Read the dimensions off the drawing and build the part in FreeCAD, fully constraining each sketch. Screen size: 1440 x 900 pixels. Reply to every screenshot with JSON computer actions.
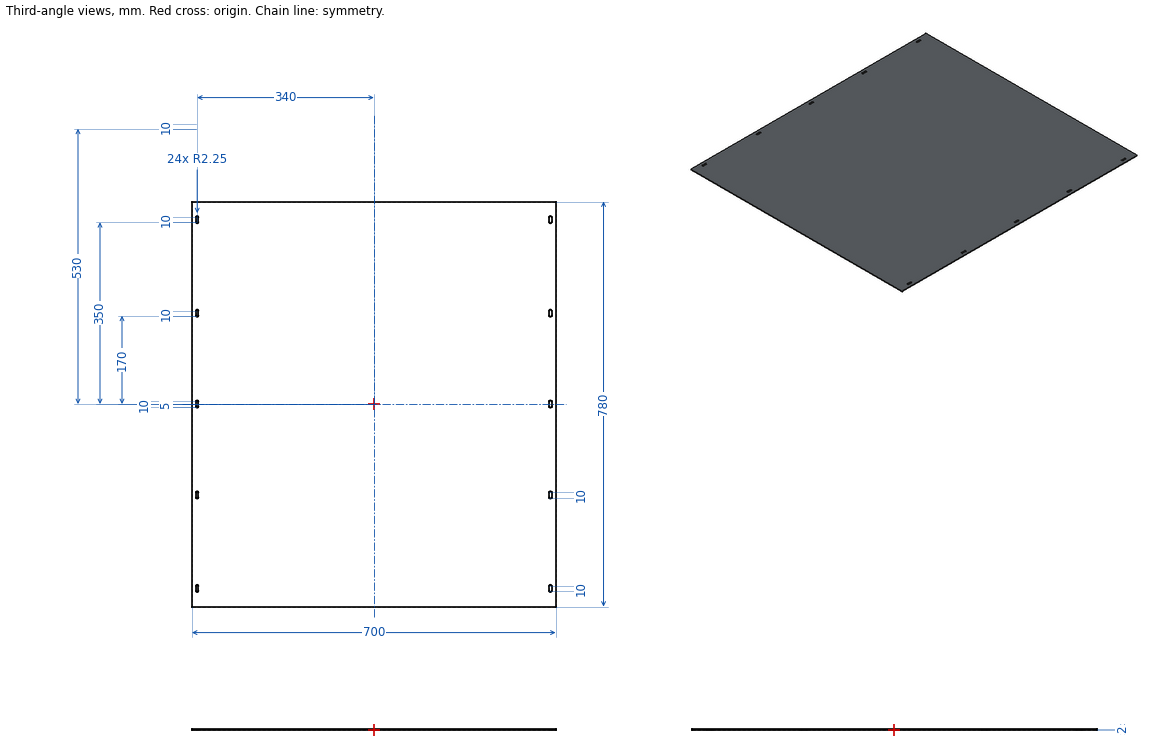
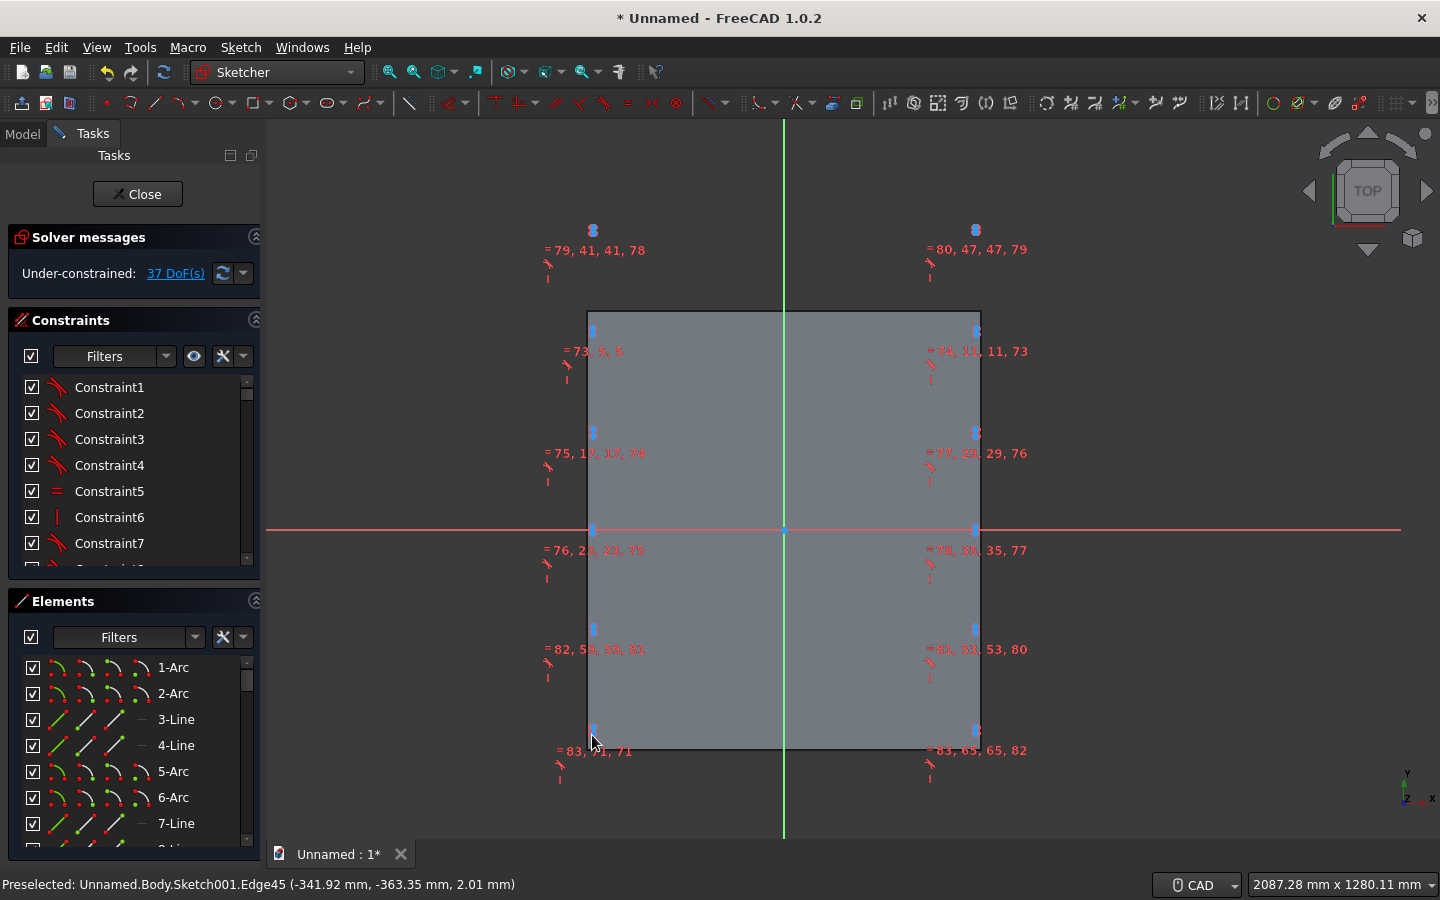
{"action": "scroll", "coordinate": [593, 335], "scroll_direction": "up", "scroll_amount": 12}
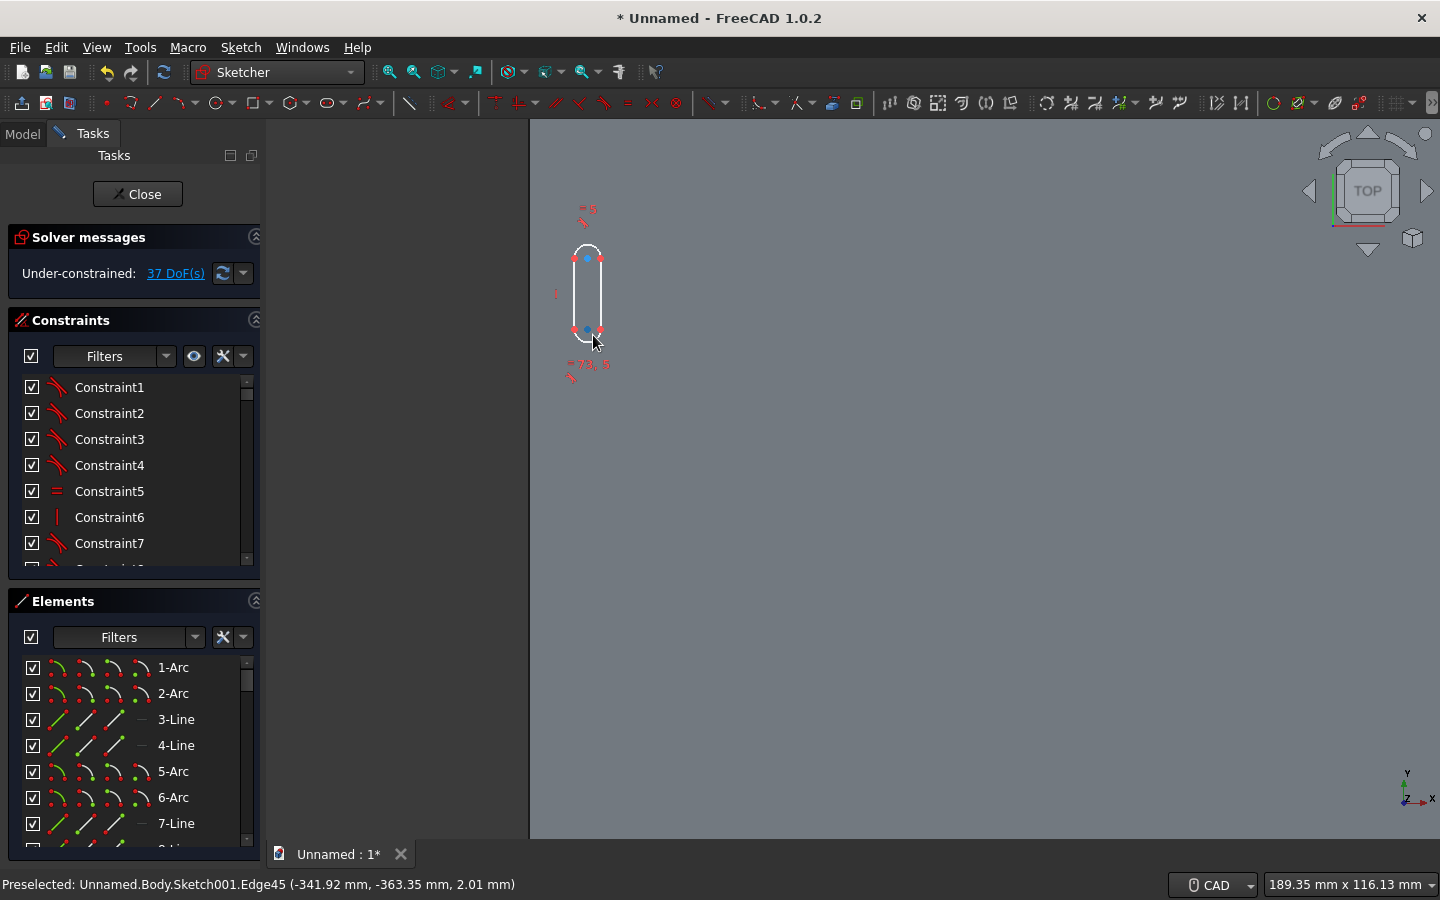
{"action": "left_click", "coordinate": [588, 329]}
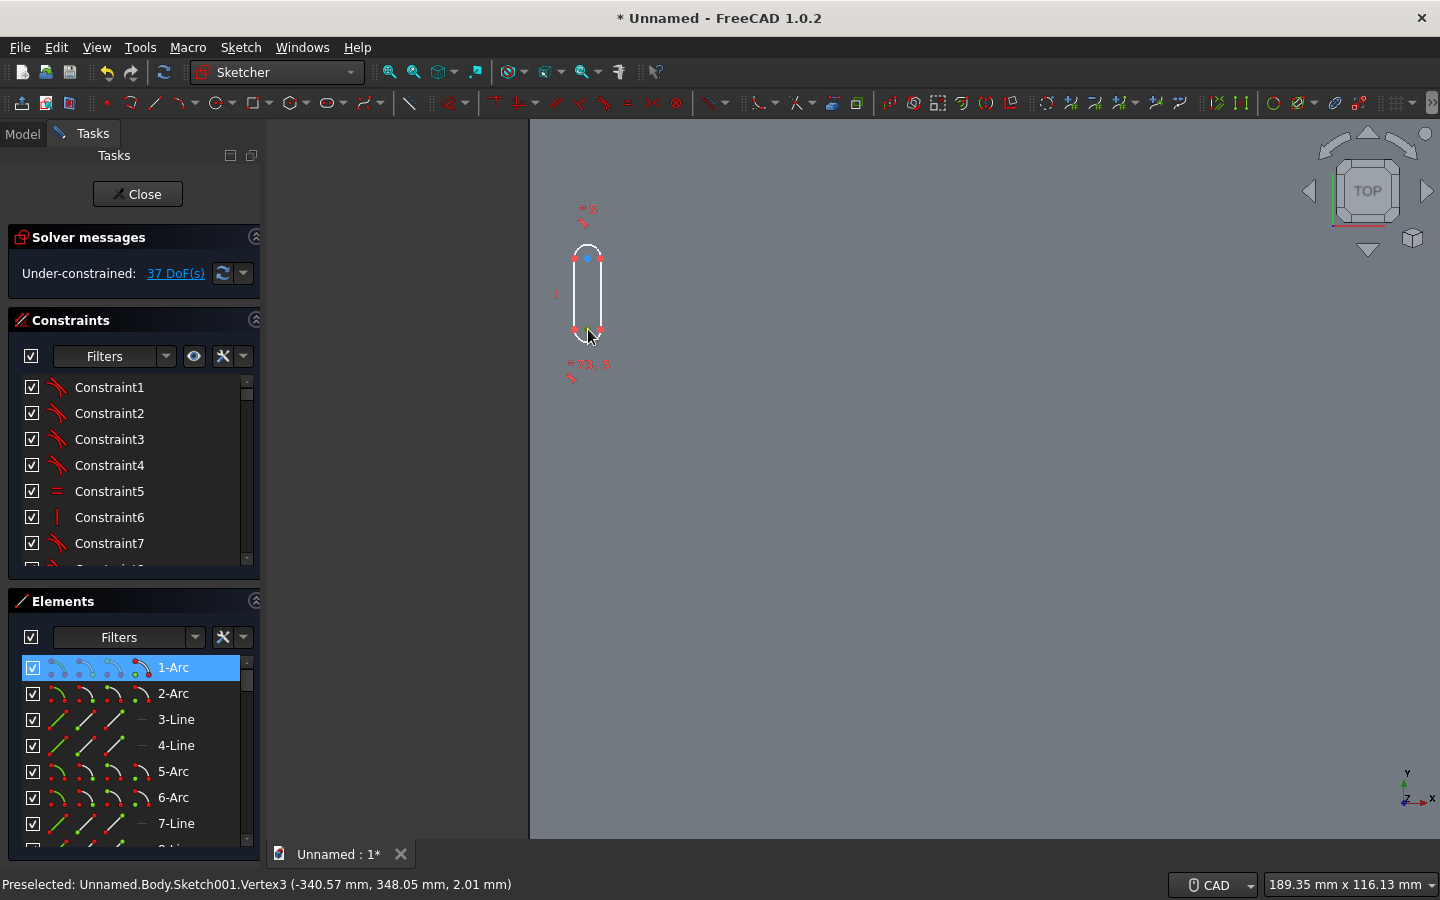
{"action": "scroll", "coordinate": [593, 334], "scroll_direction": "down", "scroll_amount": 12}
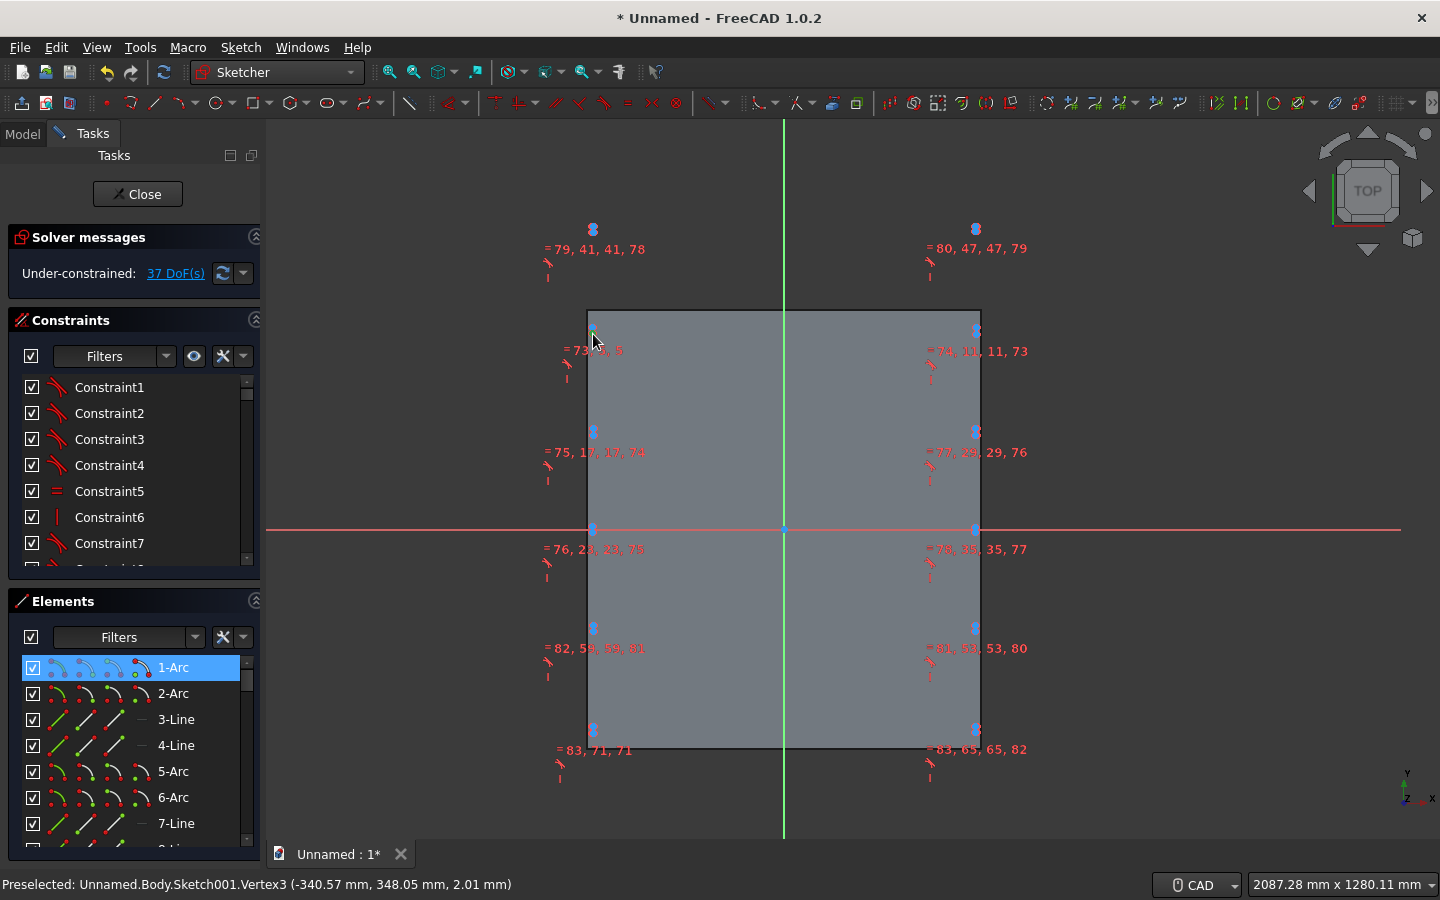
{"action": "scroll", "coordinate": [976, 334], "scroll_direction": "up", "scroll_amount": 12}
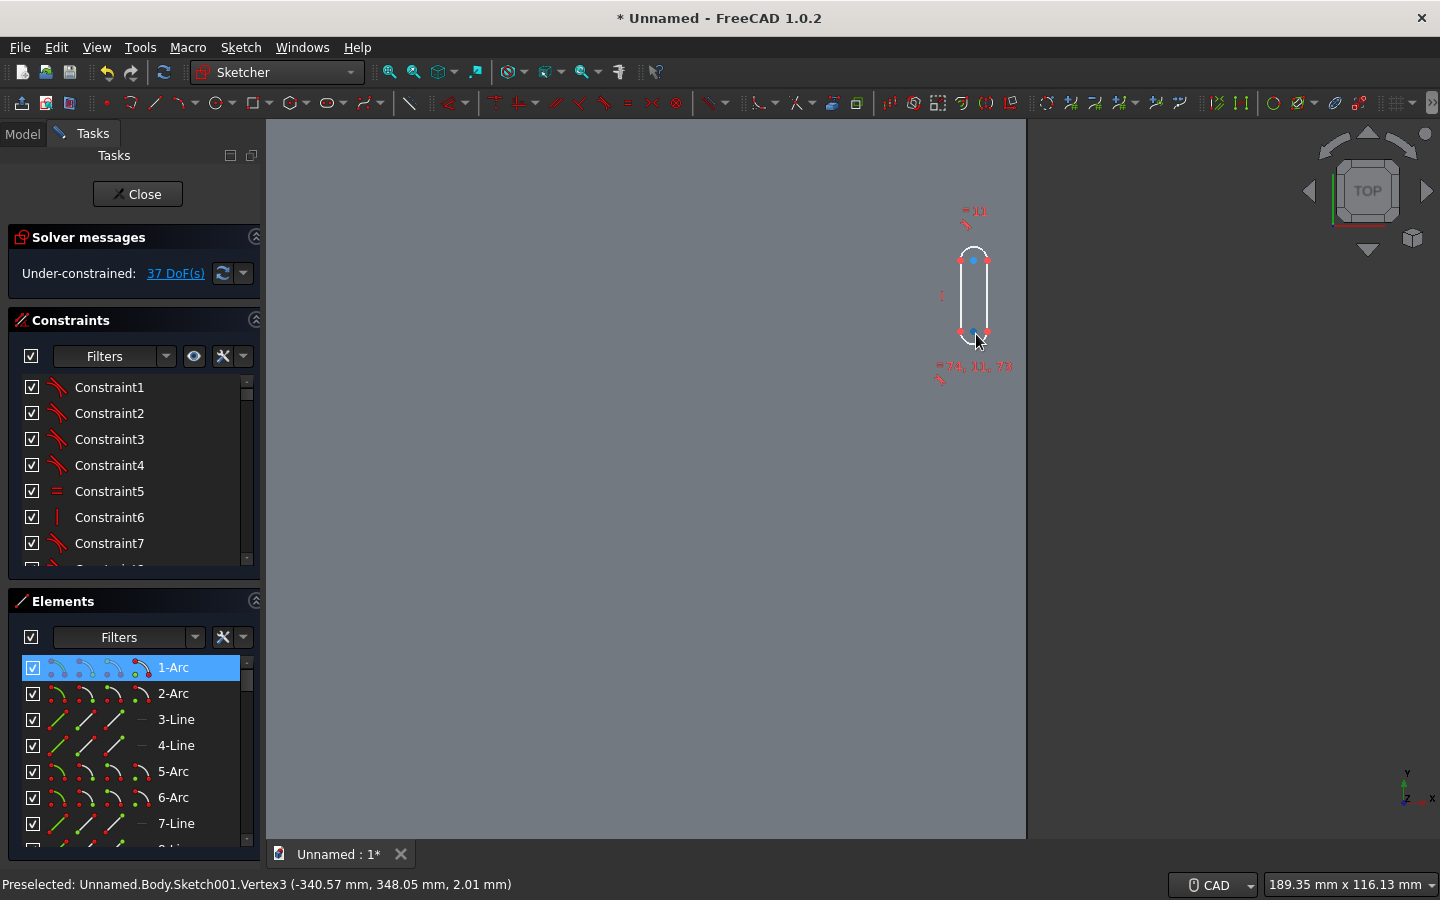
{"action": "left_click", "coordinate": [974, 331]}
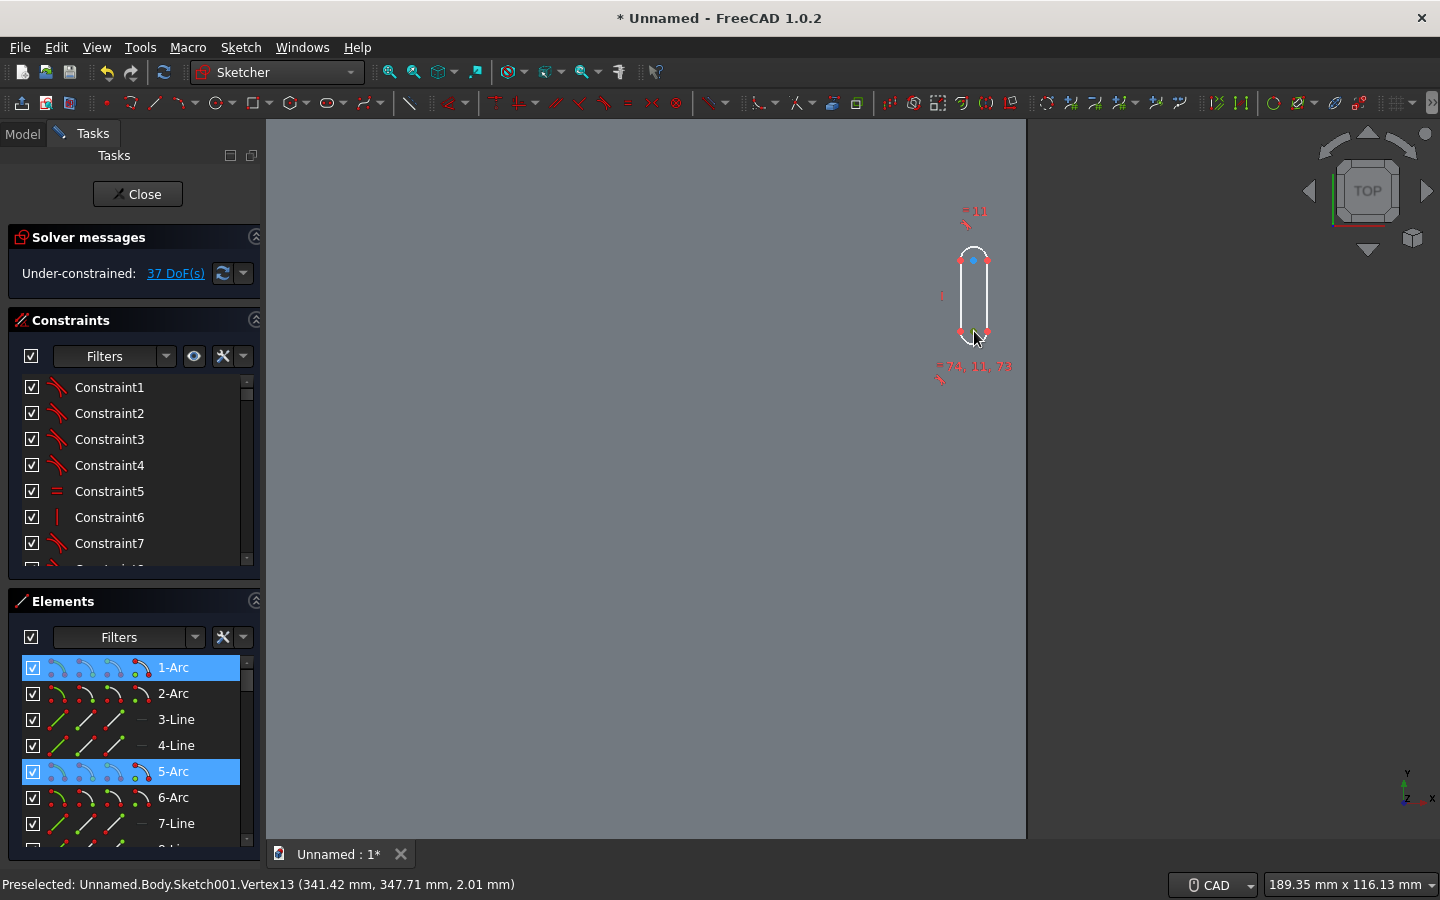
{"action": "scroll", "coordinate": [977, 334], "scroll_direction": "down", "scroll_amount": 12}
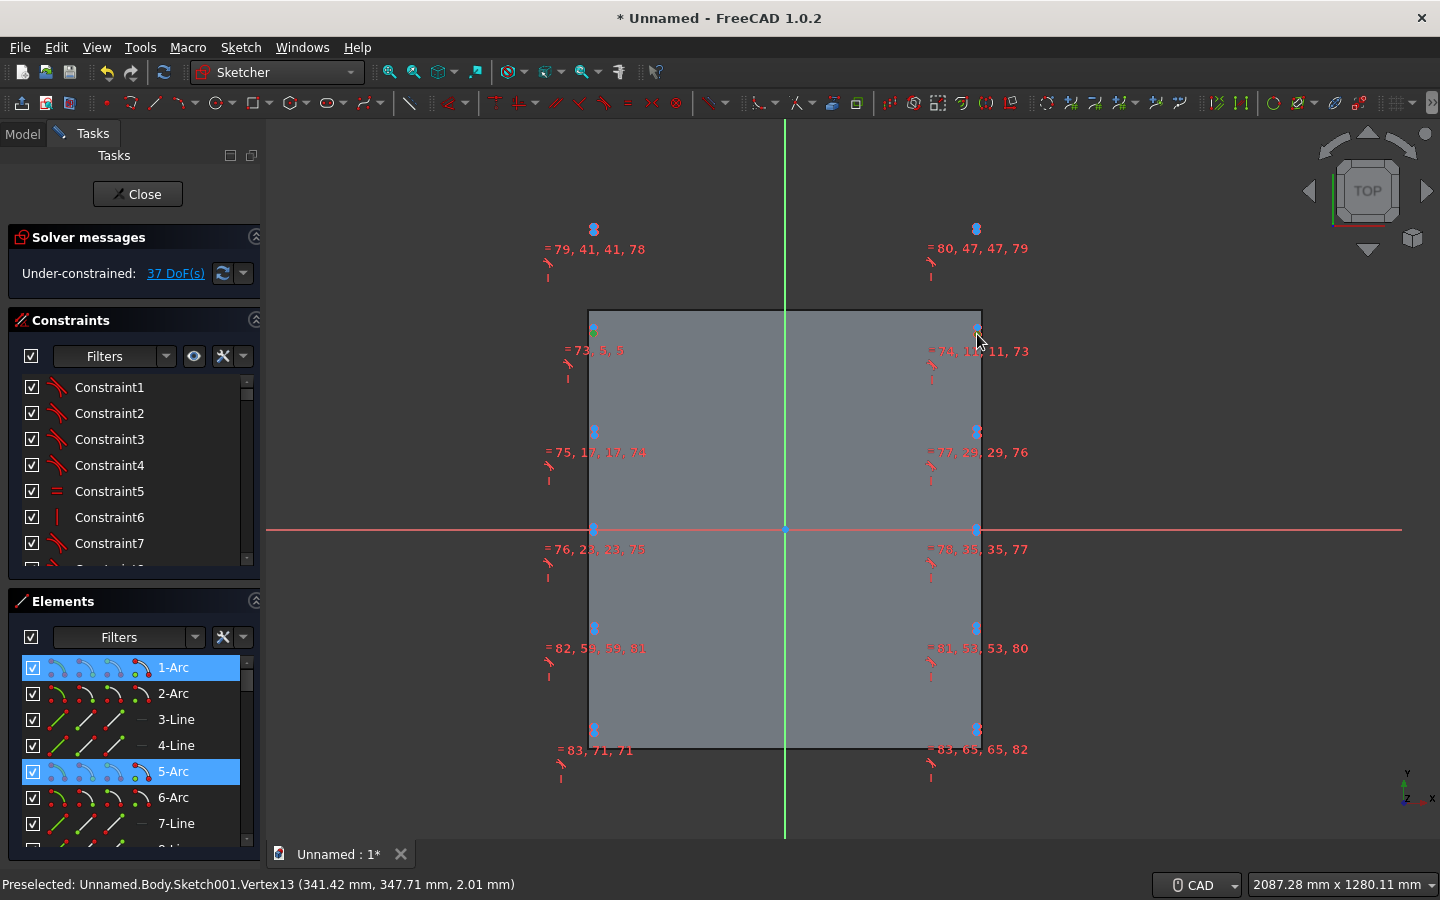
{"action": "left_click", "coordinate": [785, 764]}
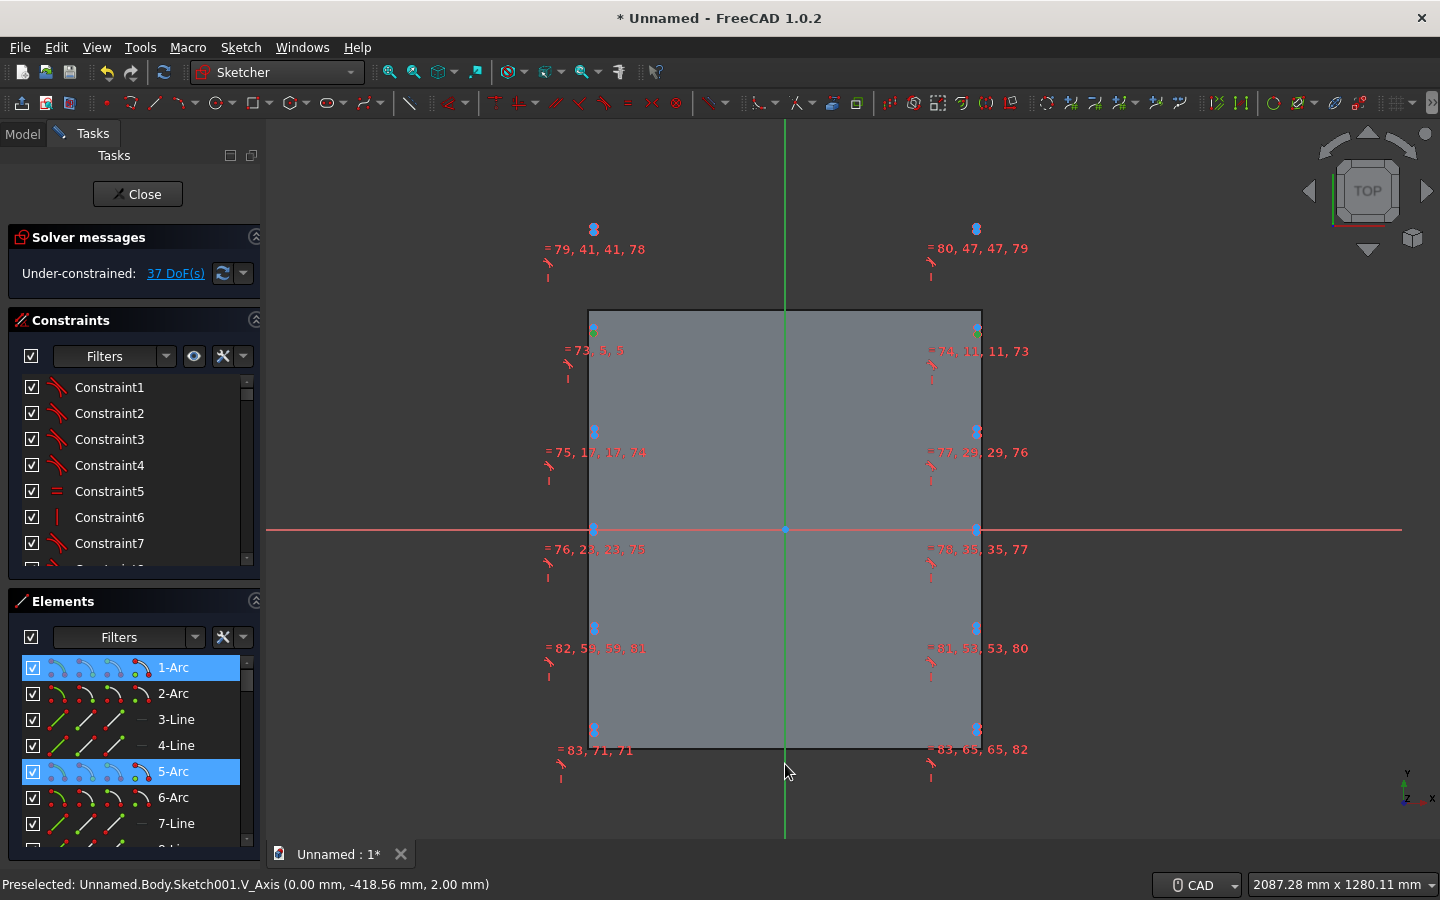
{"action": "key", "text": "s"}